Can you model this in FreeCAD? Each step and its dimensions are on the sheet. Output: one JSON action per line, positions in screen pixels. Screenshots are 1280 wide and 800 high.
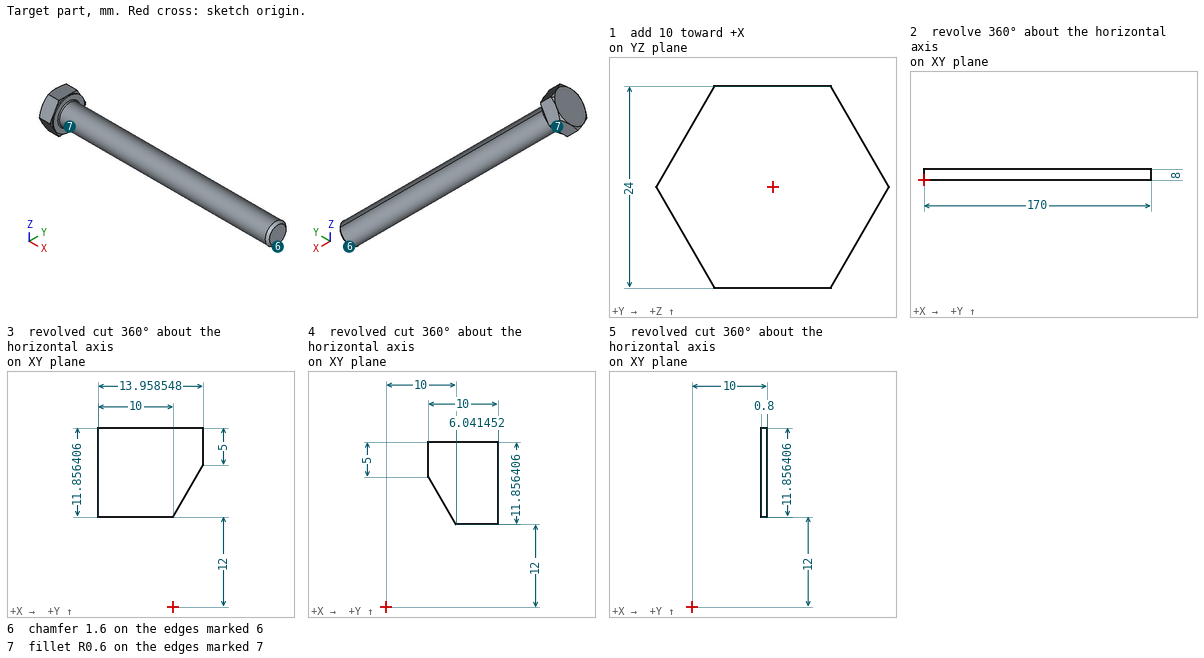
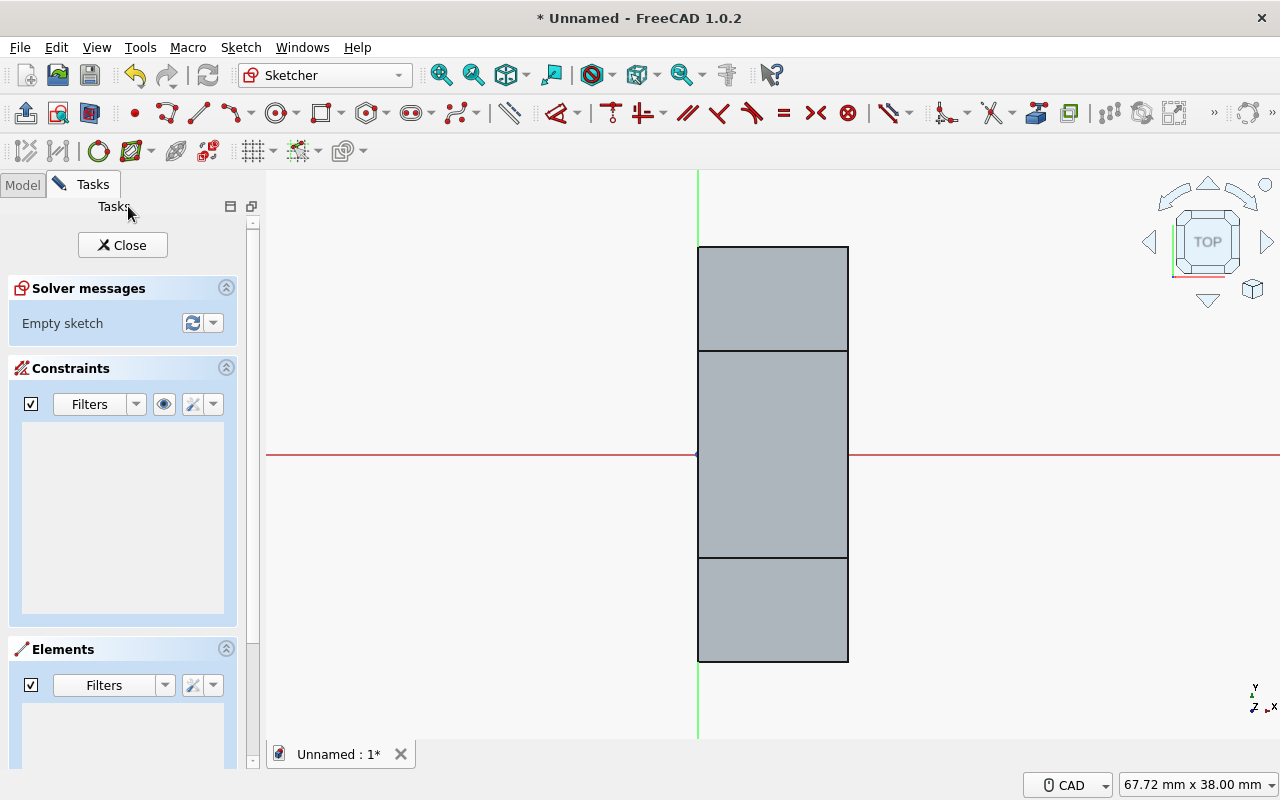
{"action": "key", "text": "q s"}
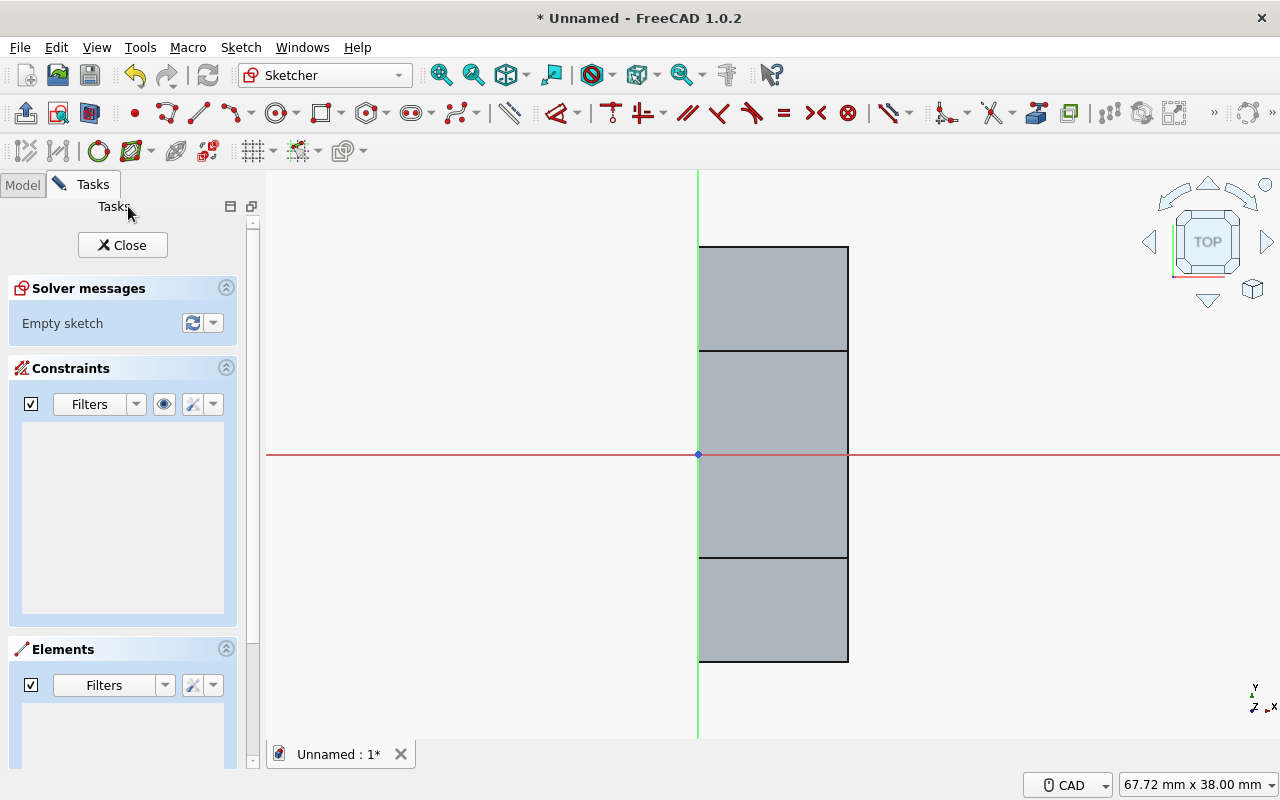
{"action": "scroll", "coordinate": [294, 474], "scroll_direction": "down", "scroll_amount": 7}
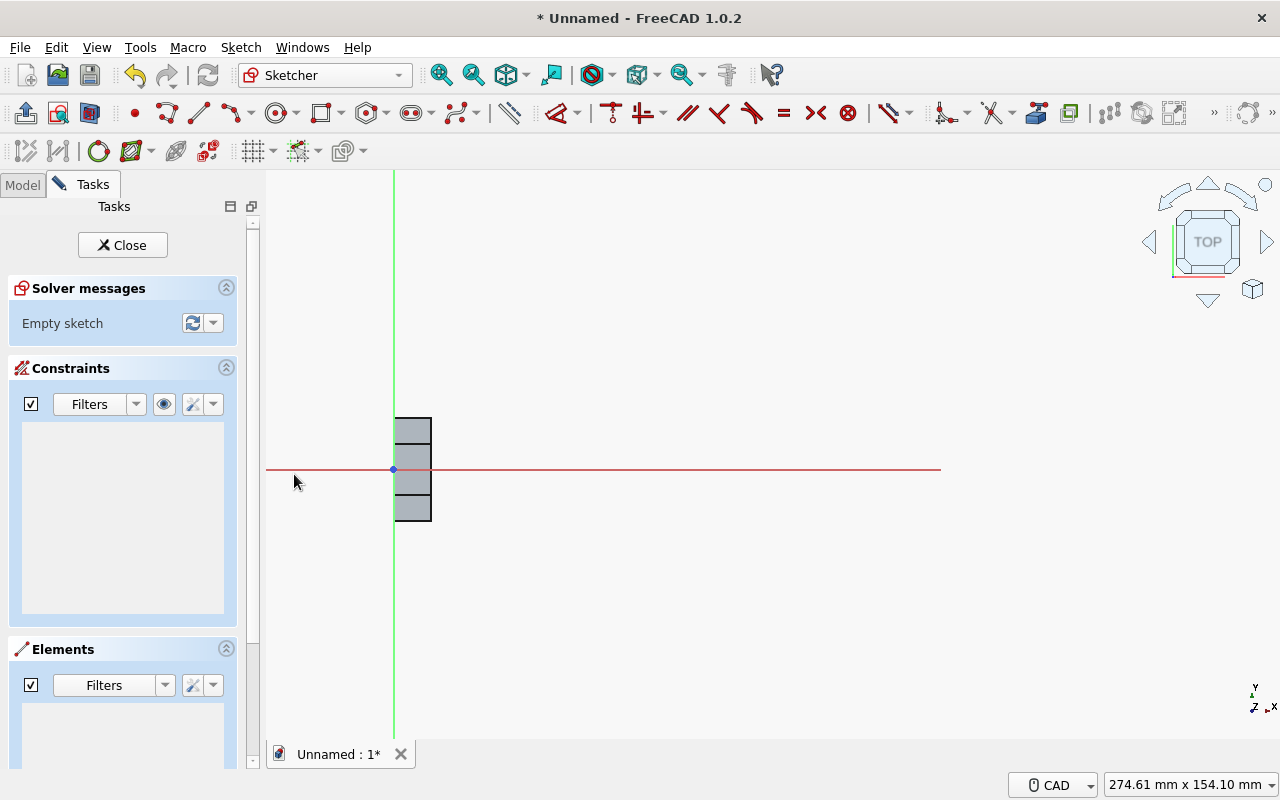
{"action": "left_click", "coordinate": [322, 114]}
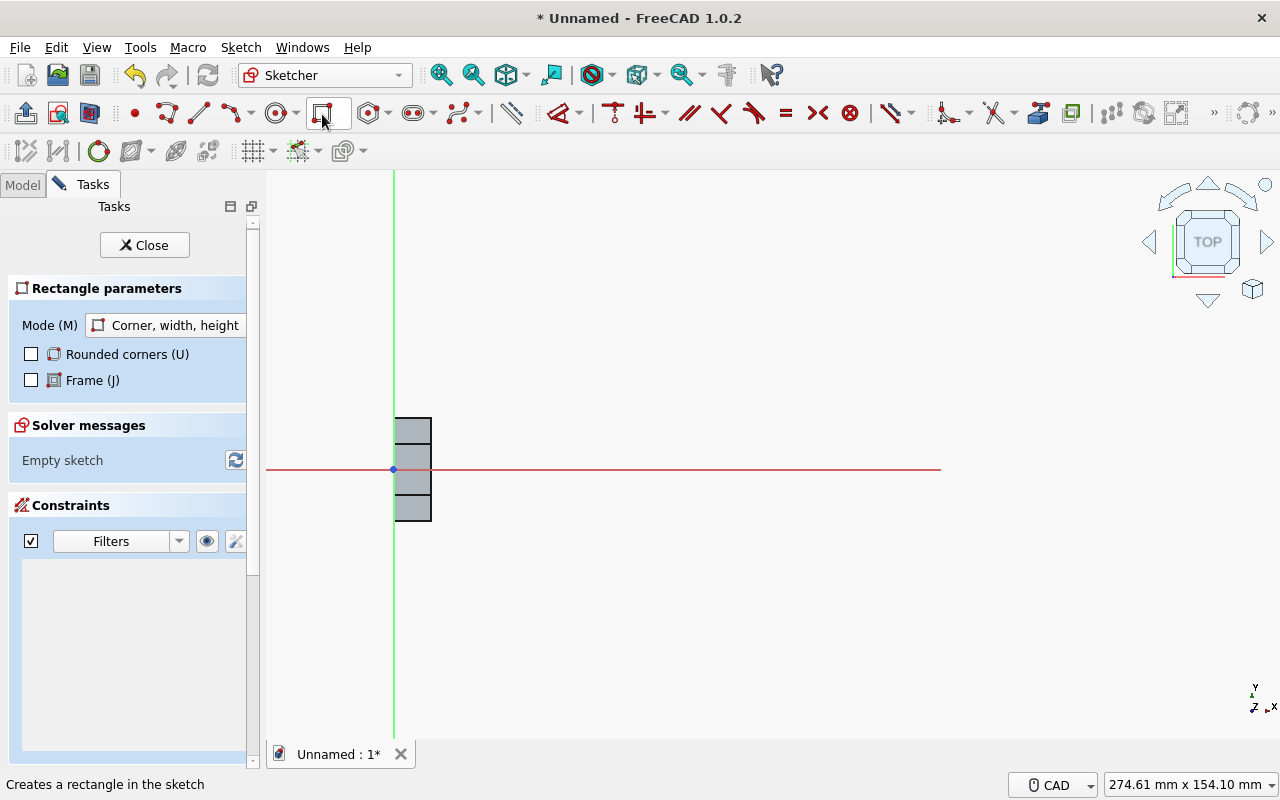
{"action": "left_click", "coordinate": [394, 470]}
{"action": "left_click", "coordinate": [1021, 440]}
{"action": "key", "text": "Escape"}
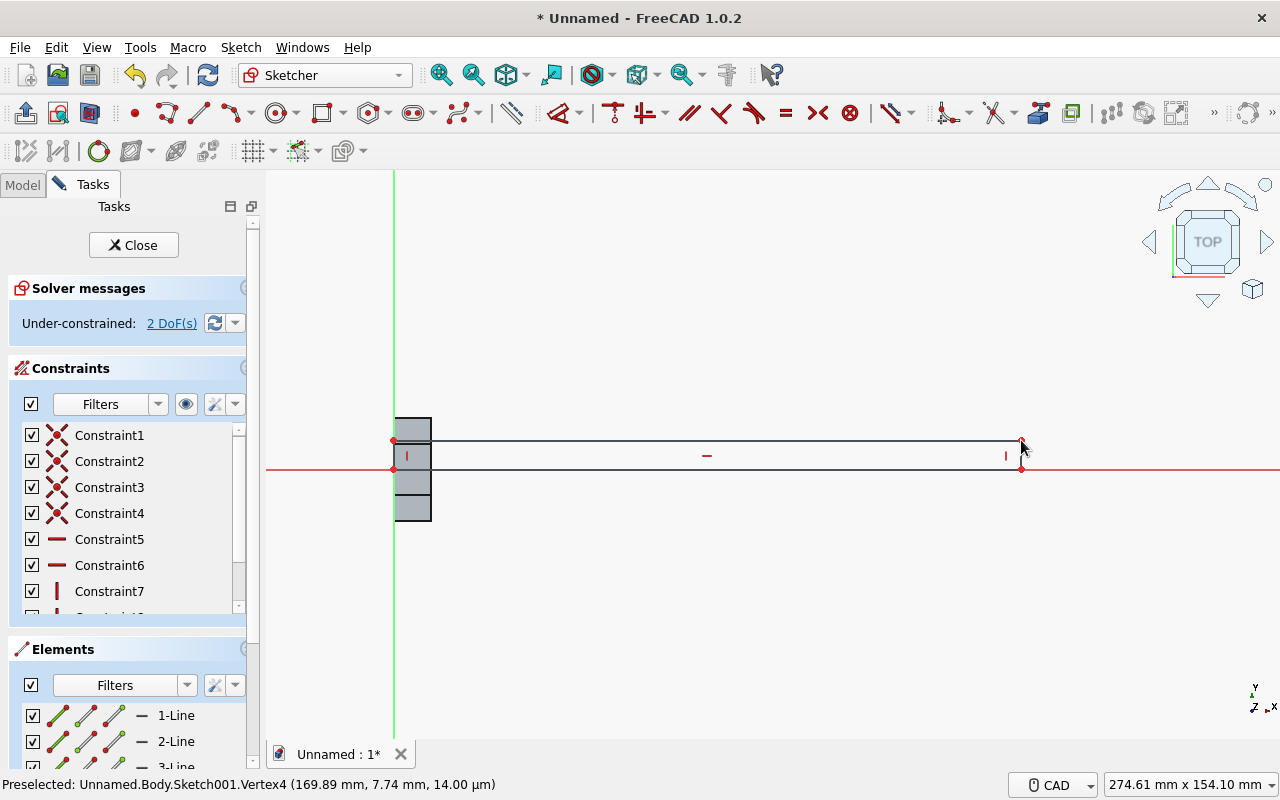
{"action": "left_click", "coordinate": [558, 114]}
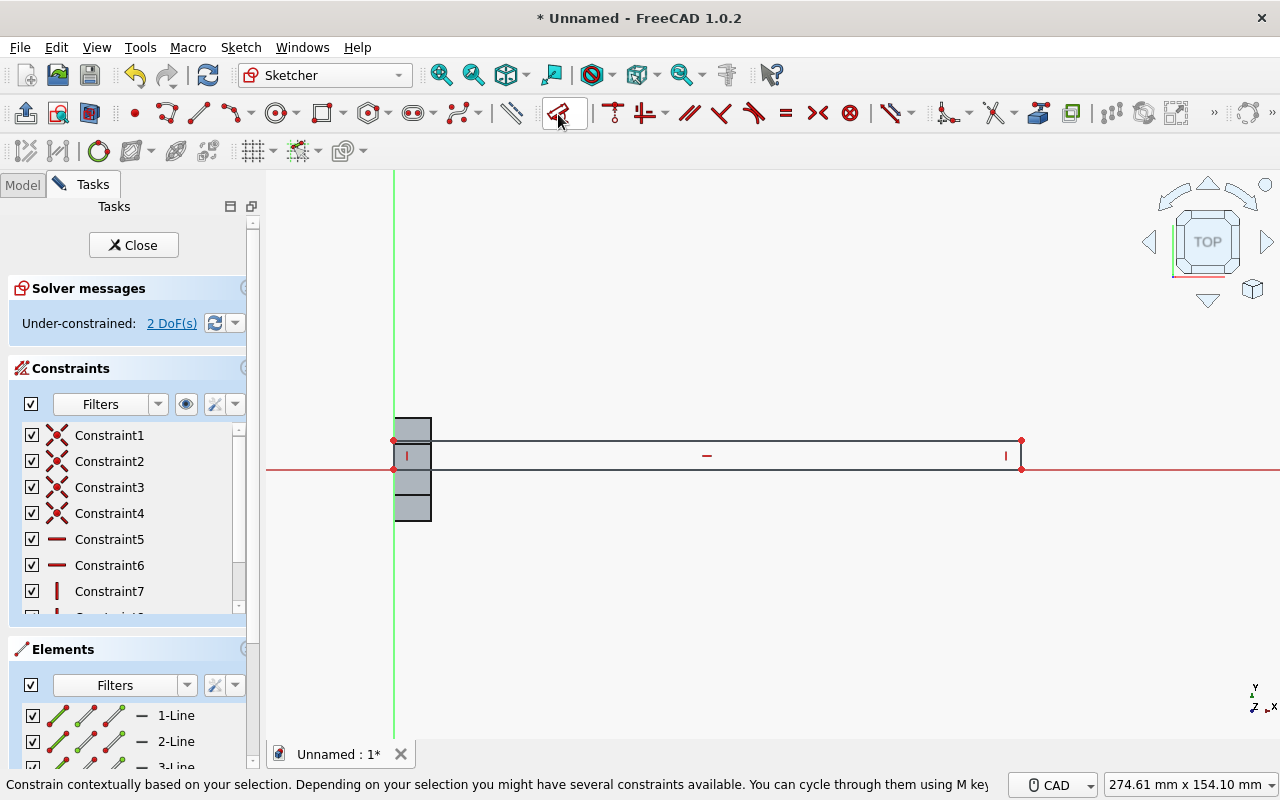
{"action": "scroll", "coordinate": [1021, 458], "scroll_direction": "up", "scroll_amount": 2}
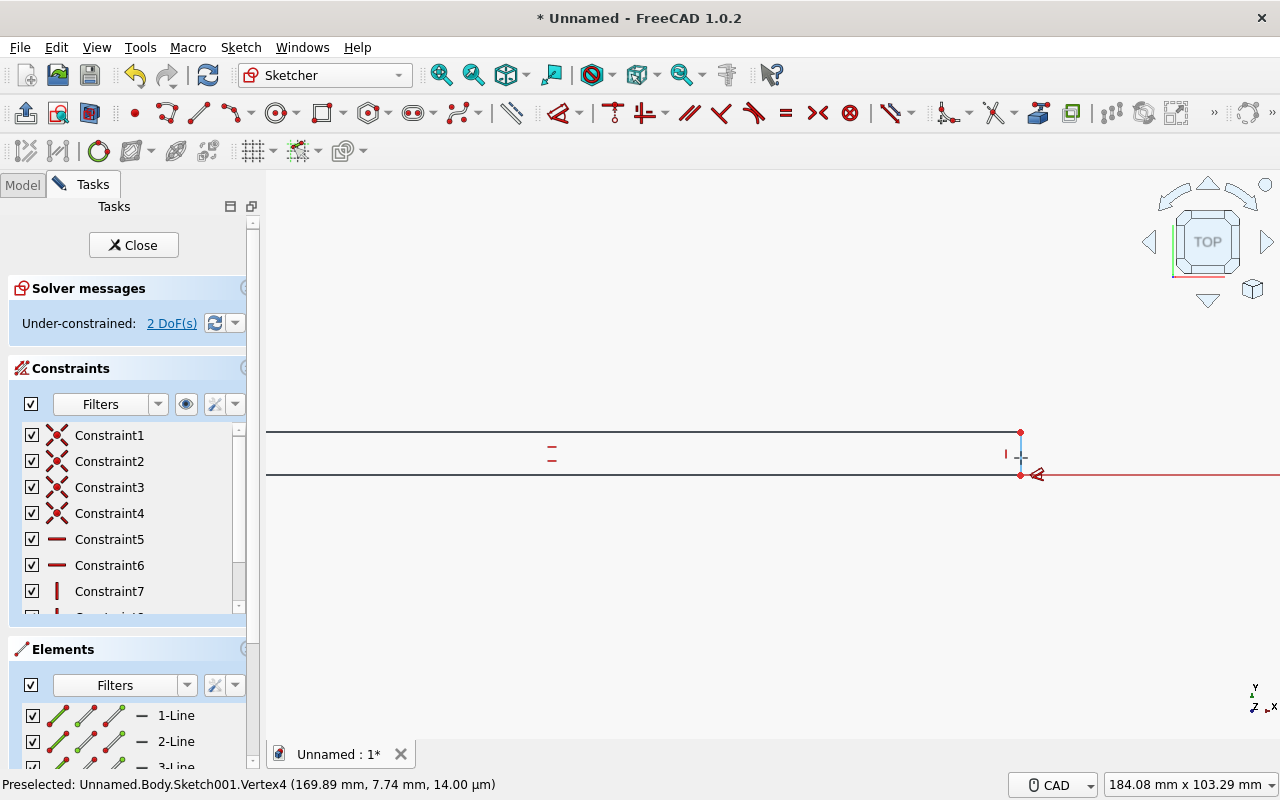
{"action": "left_click", "coordinate": [1021, 458]}
{"action": "left_click", "coordinate": [1055, 454]}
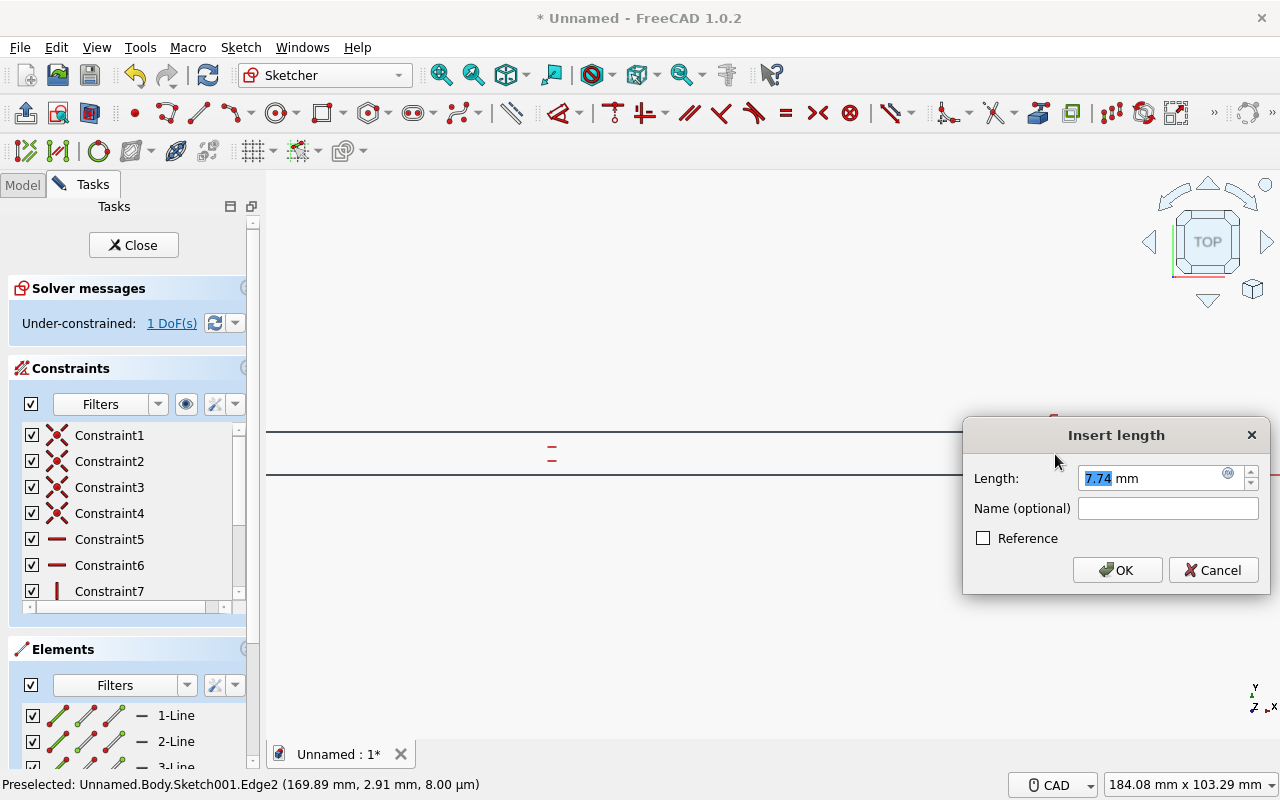
{"action": "type", "text": "8"}
{"action": "key", "text": "Return"}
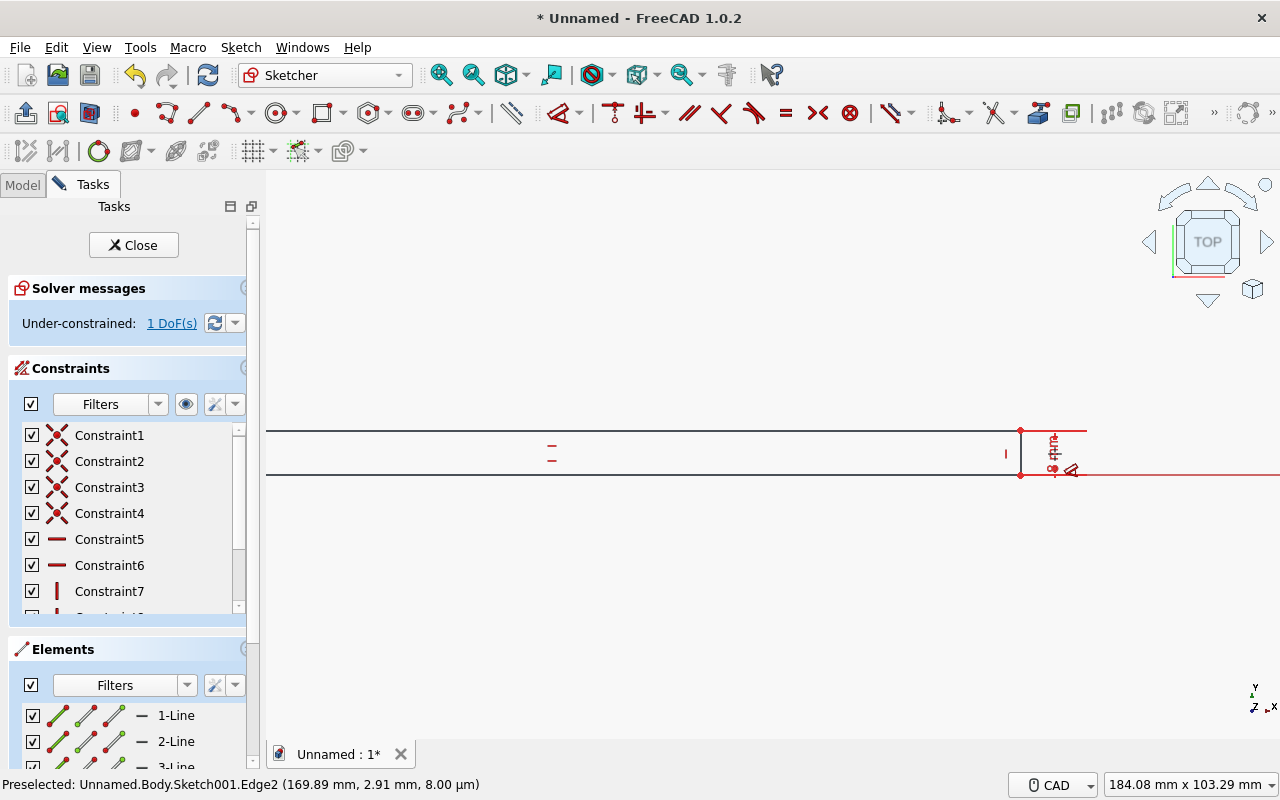
{"action": "left_click", "coordinate": [366, 475]}
{"action": "left_click", "coordinate": [657, 509]}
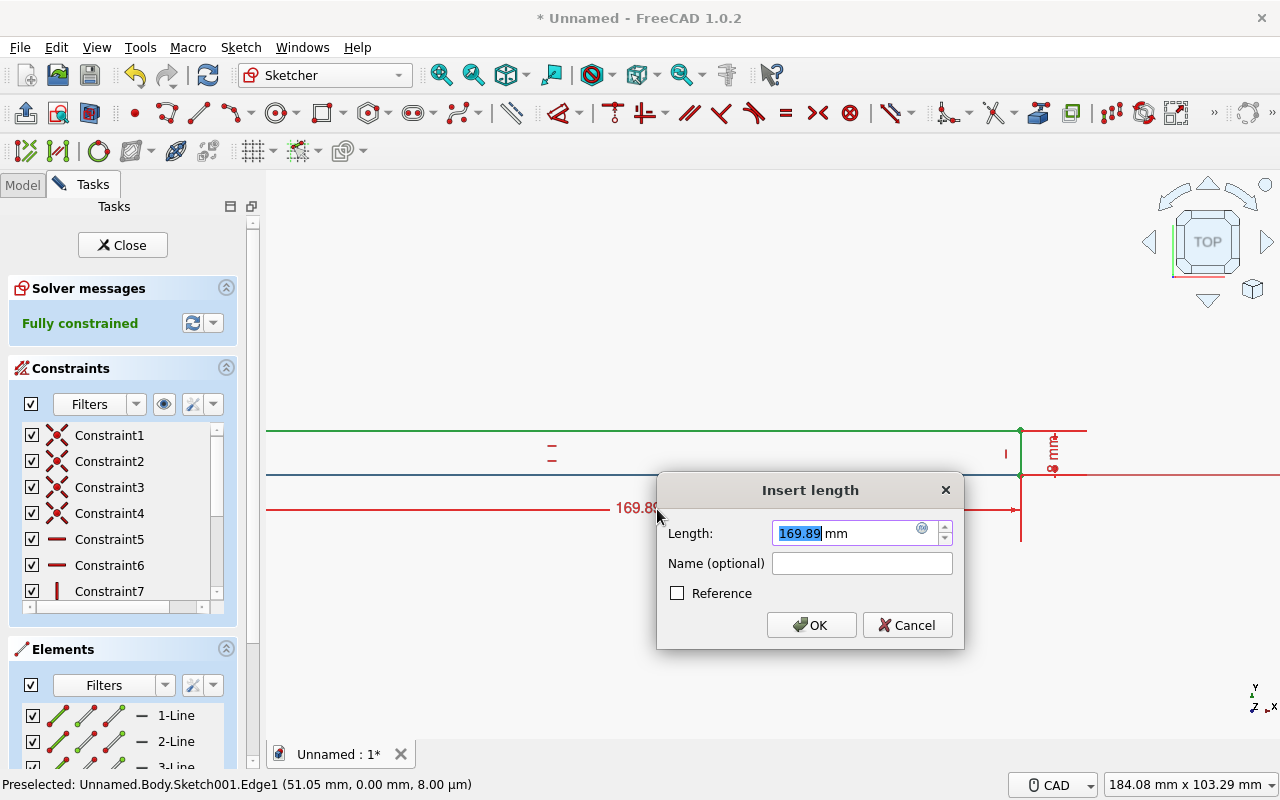
{"action": "type", "text": "170"}
{"action": "key", "text": "Return"}
{"action": "key", "text": "Escape"}